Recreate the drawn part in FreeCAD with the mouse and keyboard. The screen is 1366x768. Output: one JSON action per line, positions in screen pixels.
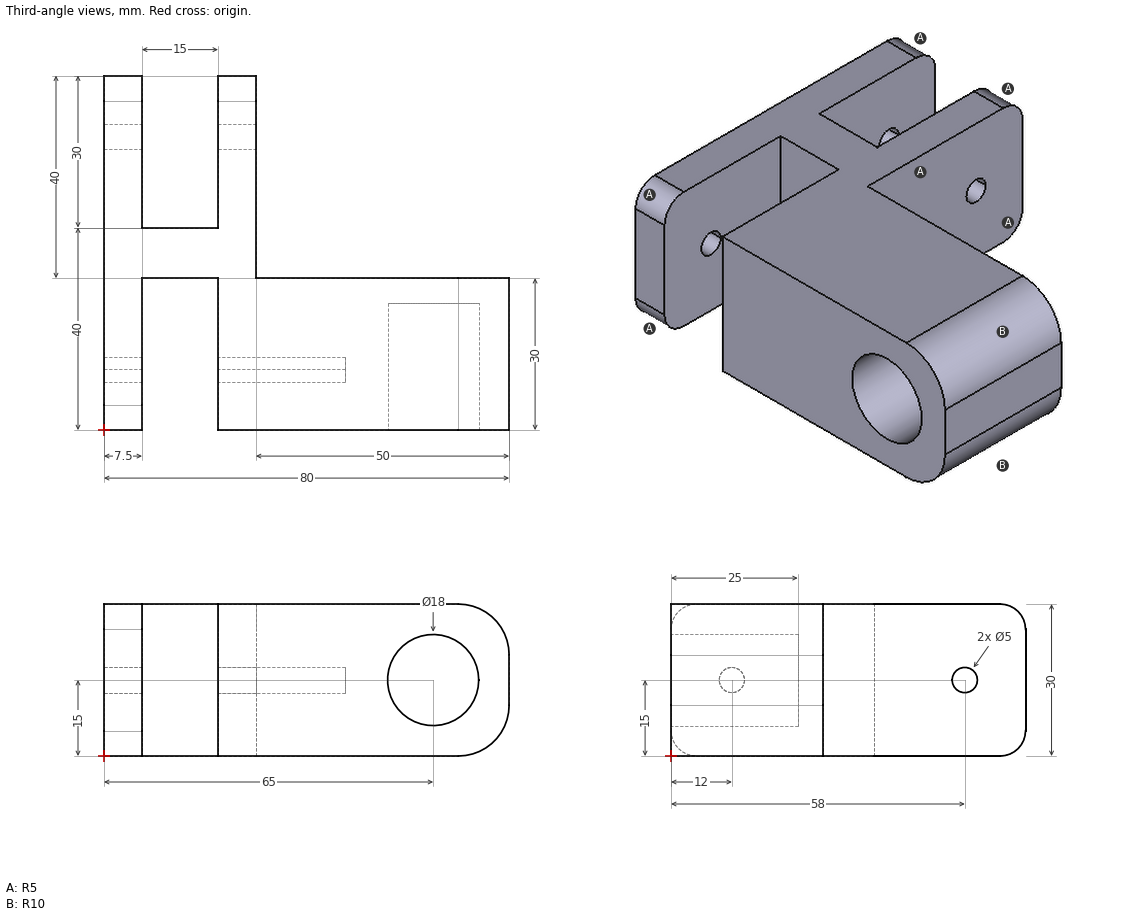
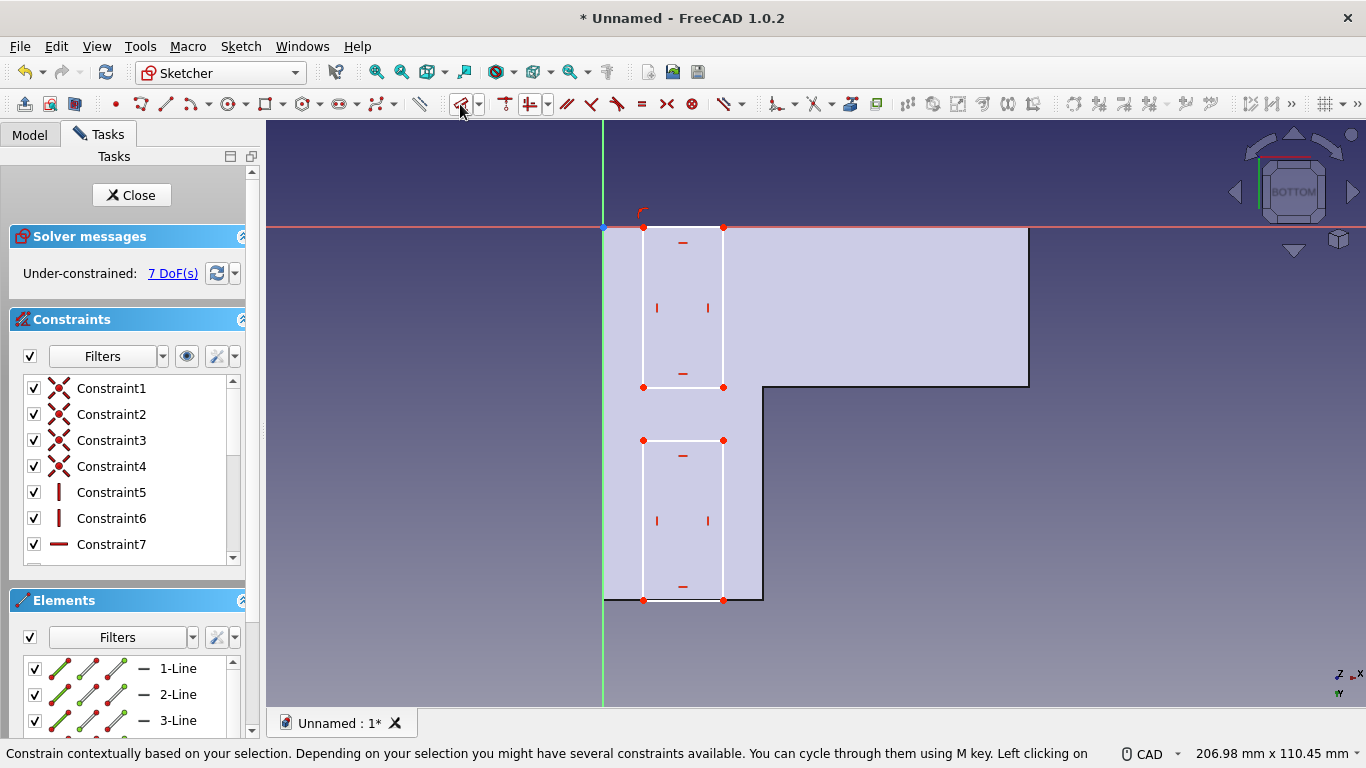
{"action": "left_click", "coordinate": [643, 489]}
{"action": "left_click", "coordinate": [677, 521]}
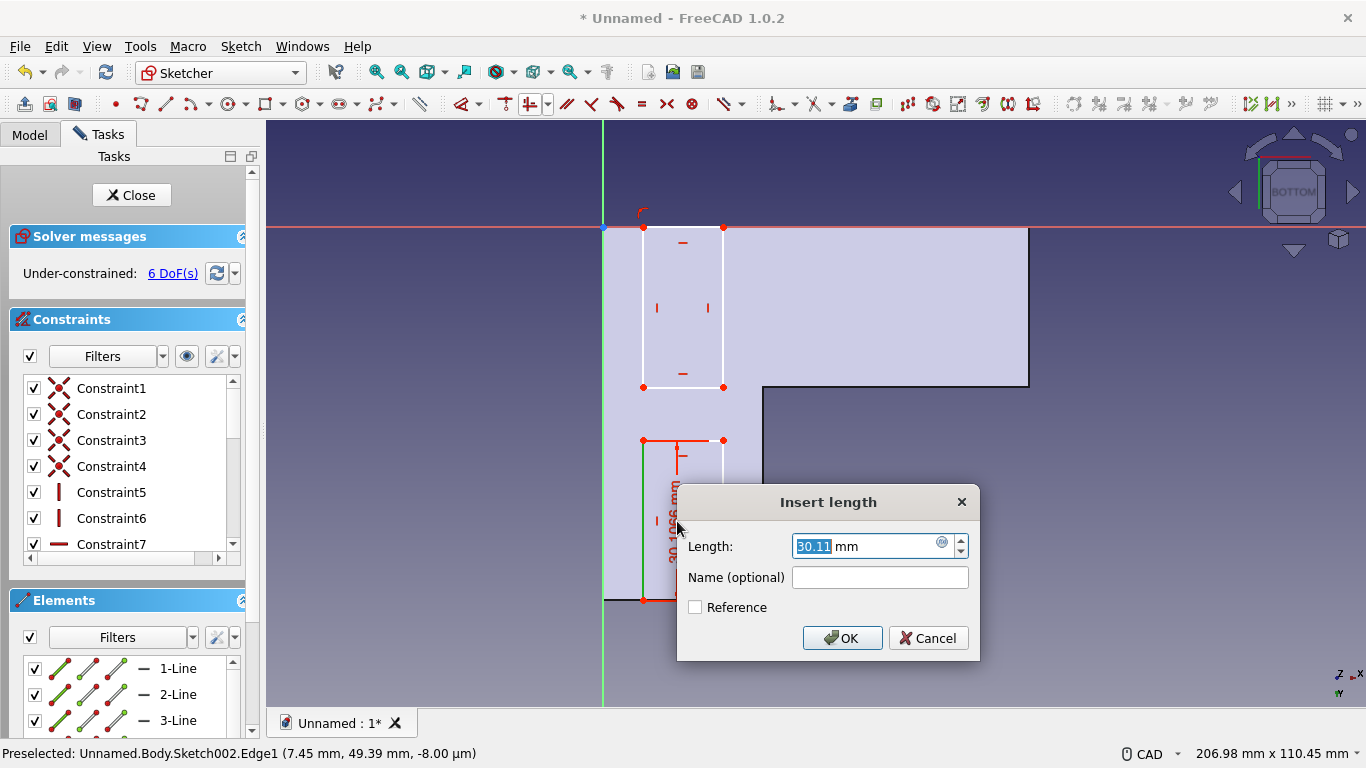
{"action": "type", "text": "30"}
{"action": "key", "text": "Return"}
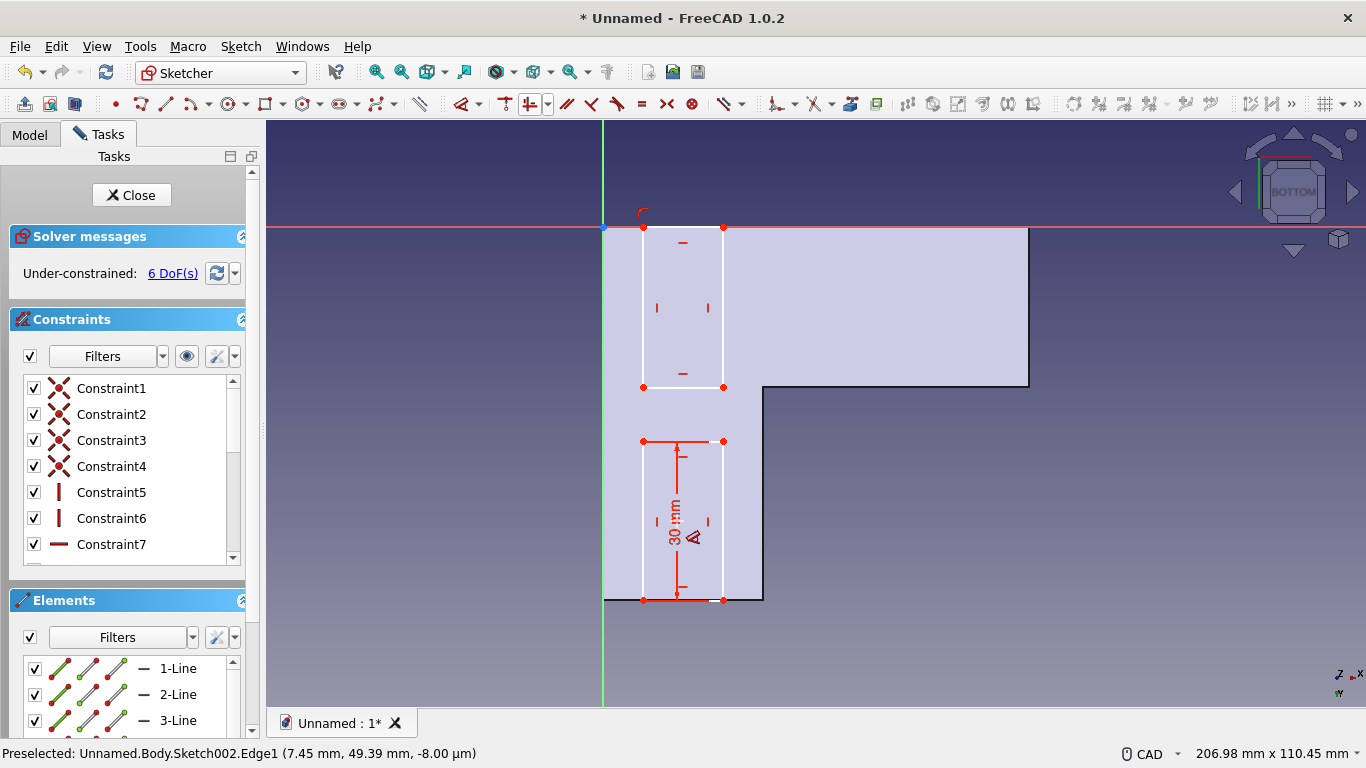
{"action": "left_click", "coordinate": [667, 601]}
{"action": "left_click", "coordinate": [683, 635]}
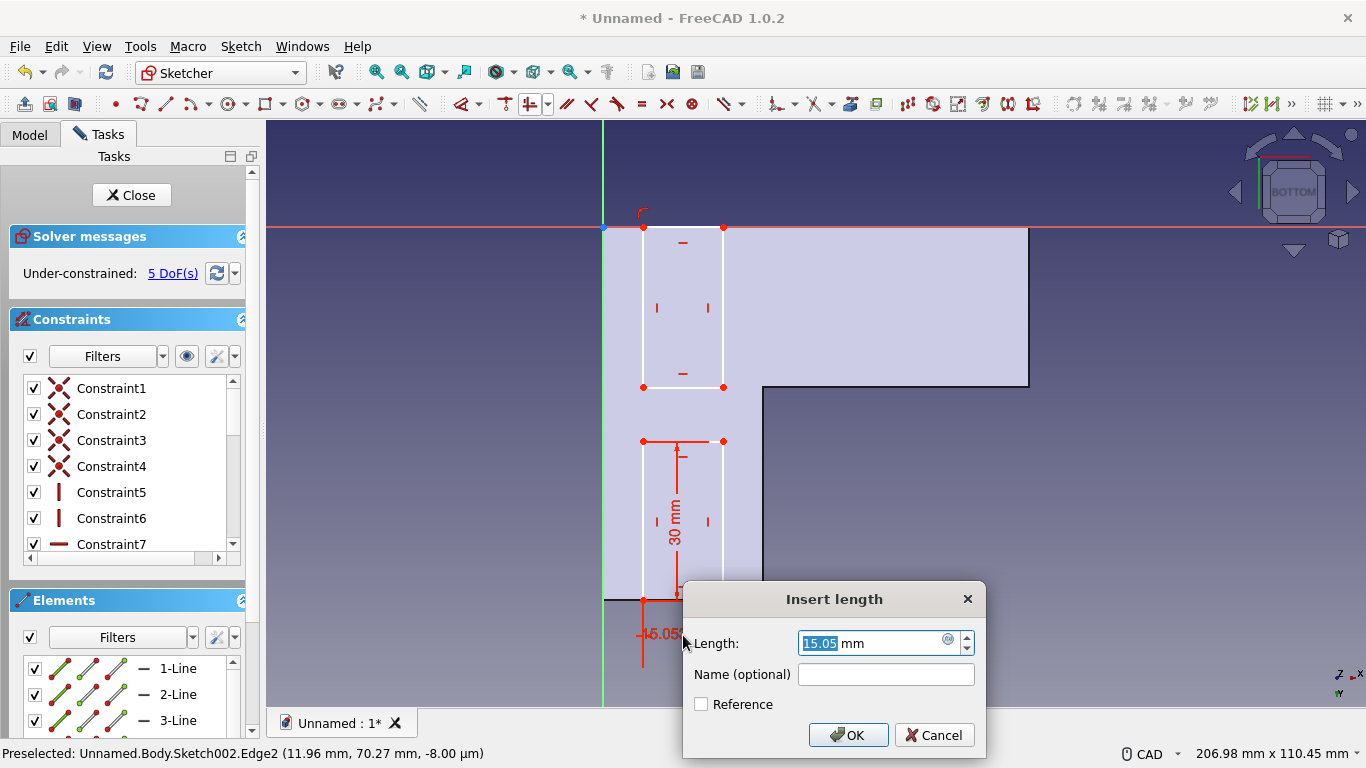
{"action": "type", "text": "15"}
{"action": "key", "text": "Return"}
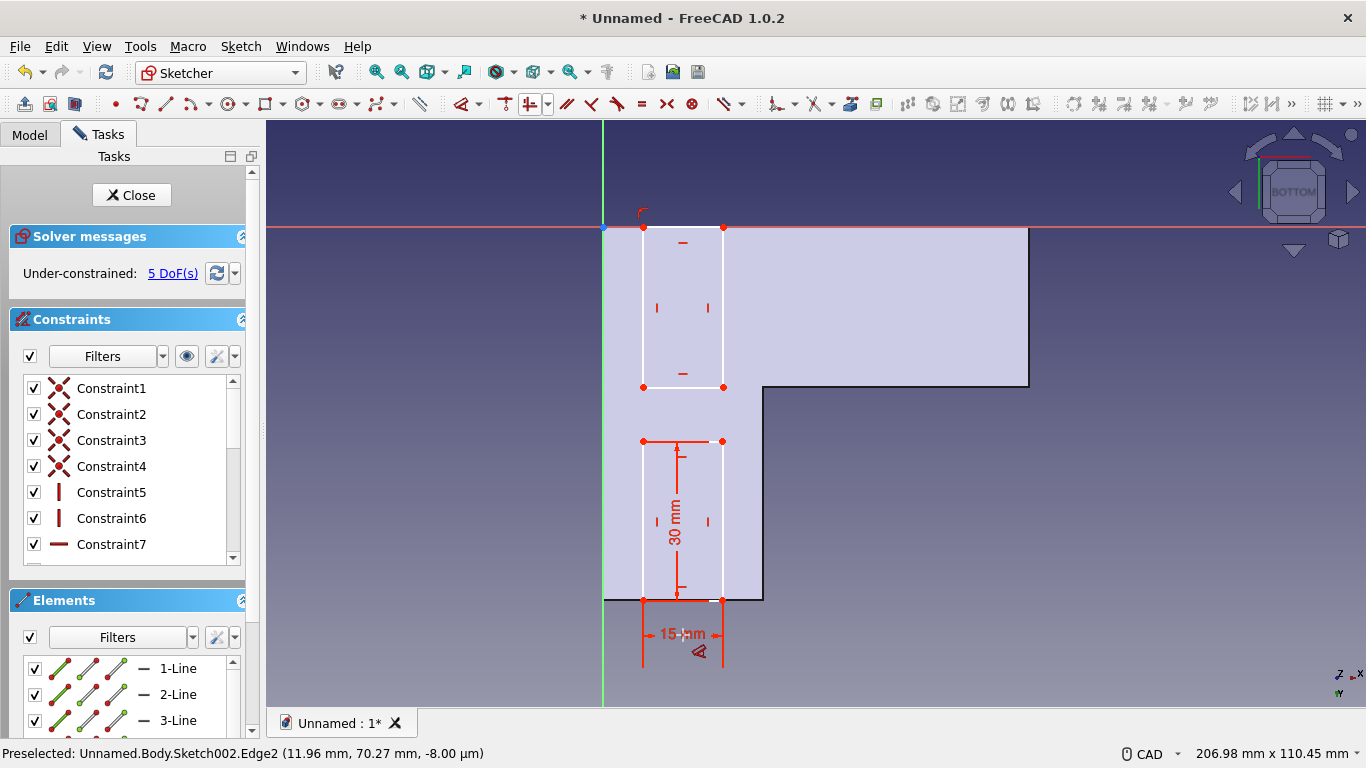
{"action": "left_click", "coordinate": [643, 276]}
{"action": "left_click", "coordinate": [677, 308]}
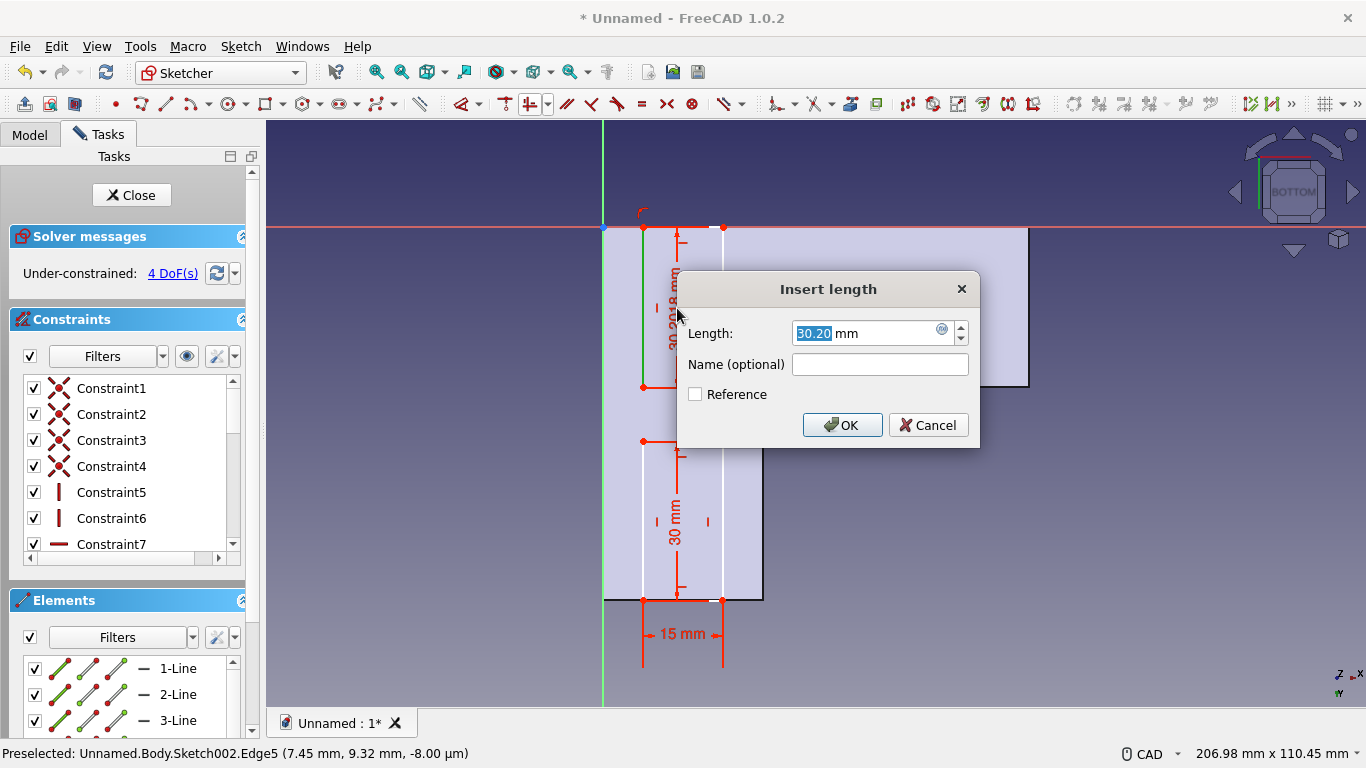
{"action": "type", "text": "30"}
{"action": "key", "text": "Return"}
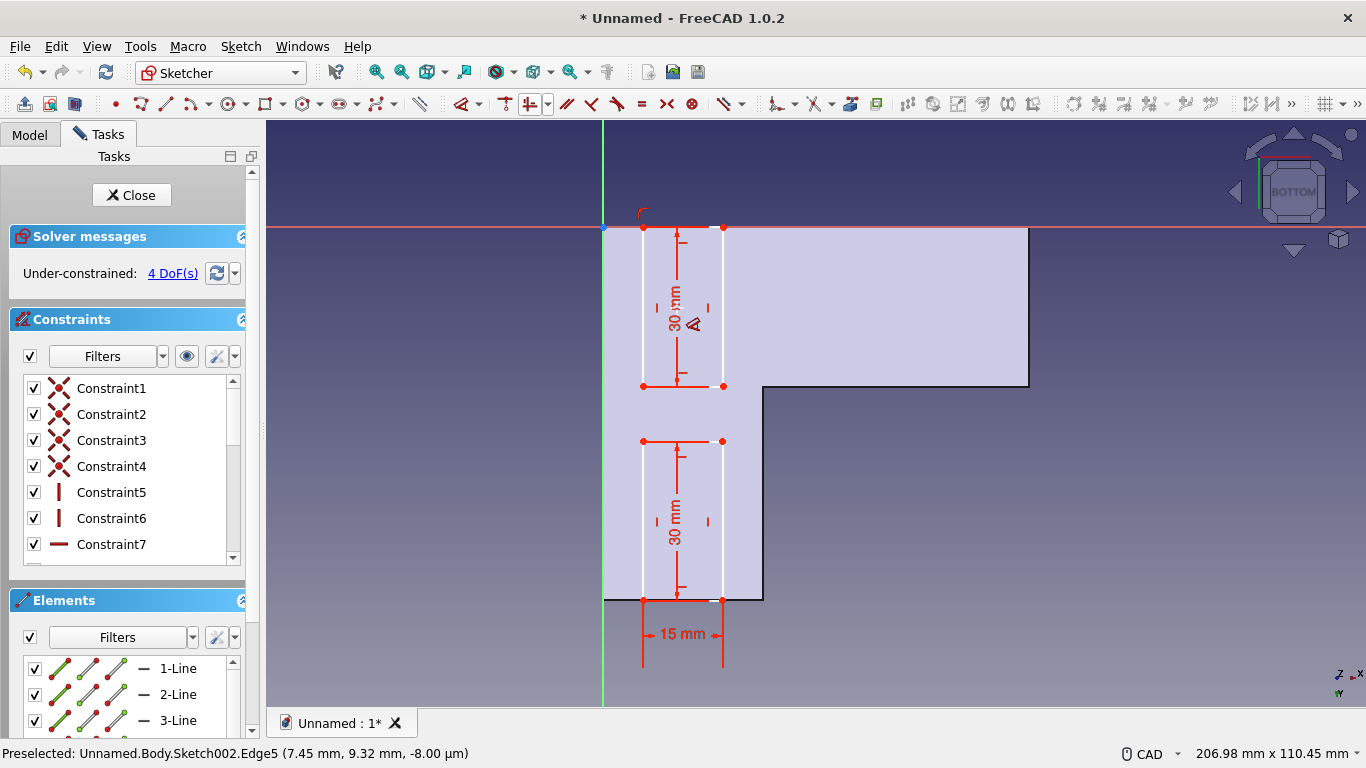
{"action": "left_click", "coordinate": [667, 387]}
{"action": "left_click", "coordinate": [683, 353]}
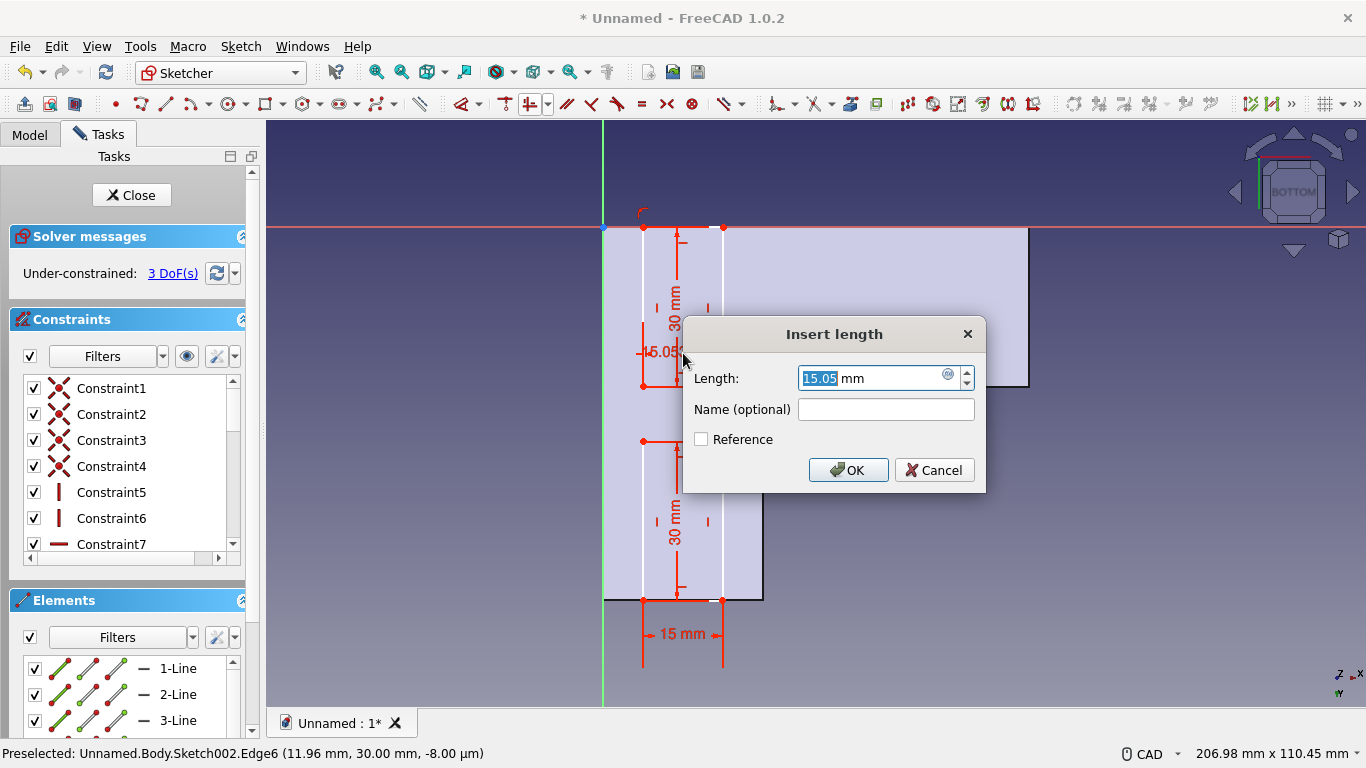
{"action": "type", "text": "15"}
{"action": "key", "text": "Return"}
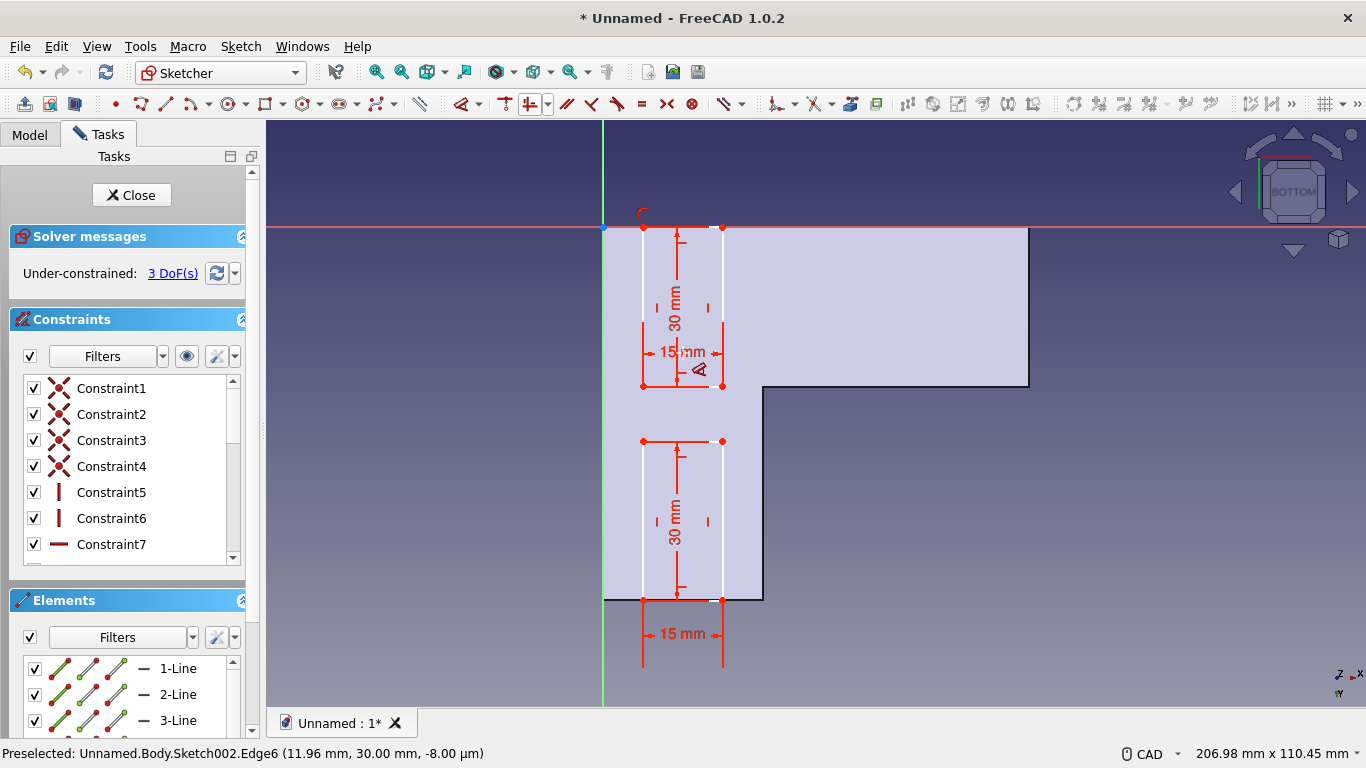
{"action": "left_click", "coordinate": [643, 442]}
{"action": "left_click", "coordinate": [569, 335]}